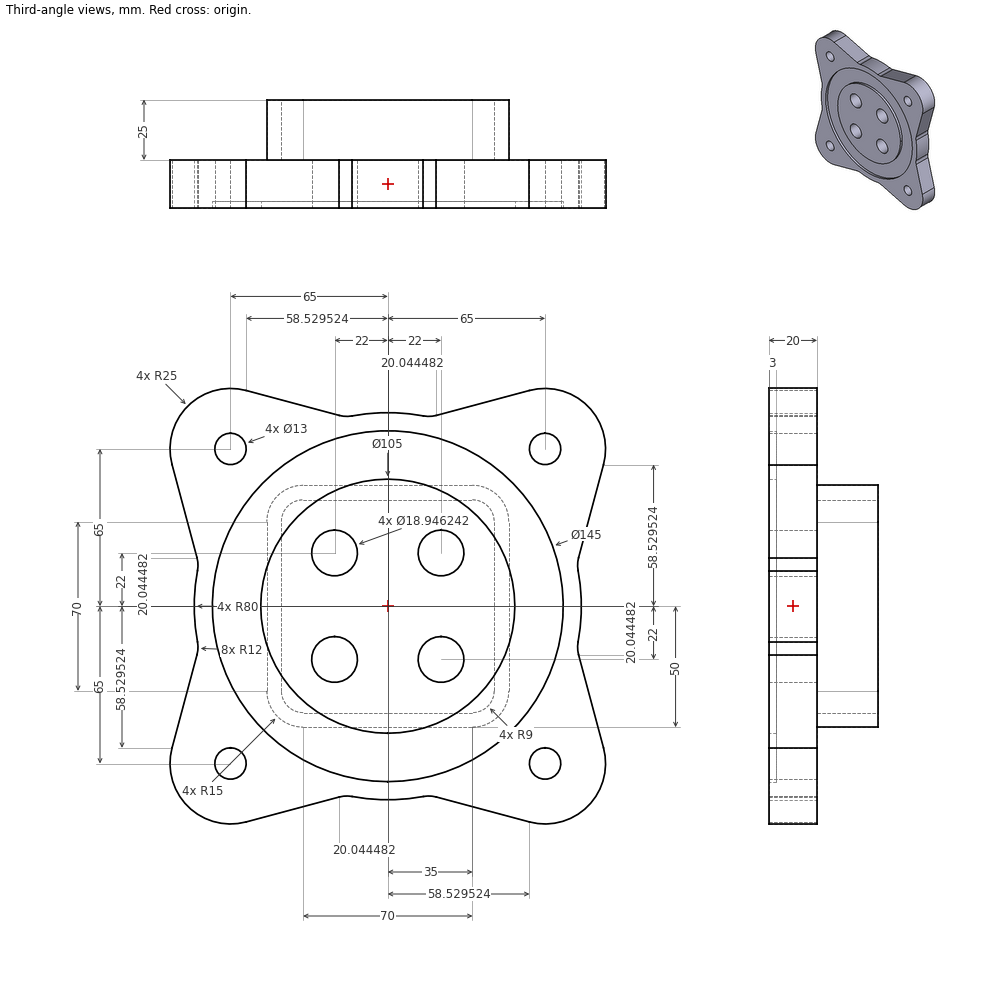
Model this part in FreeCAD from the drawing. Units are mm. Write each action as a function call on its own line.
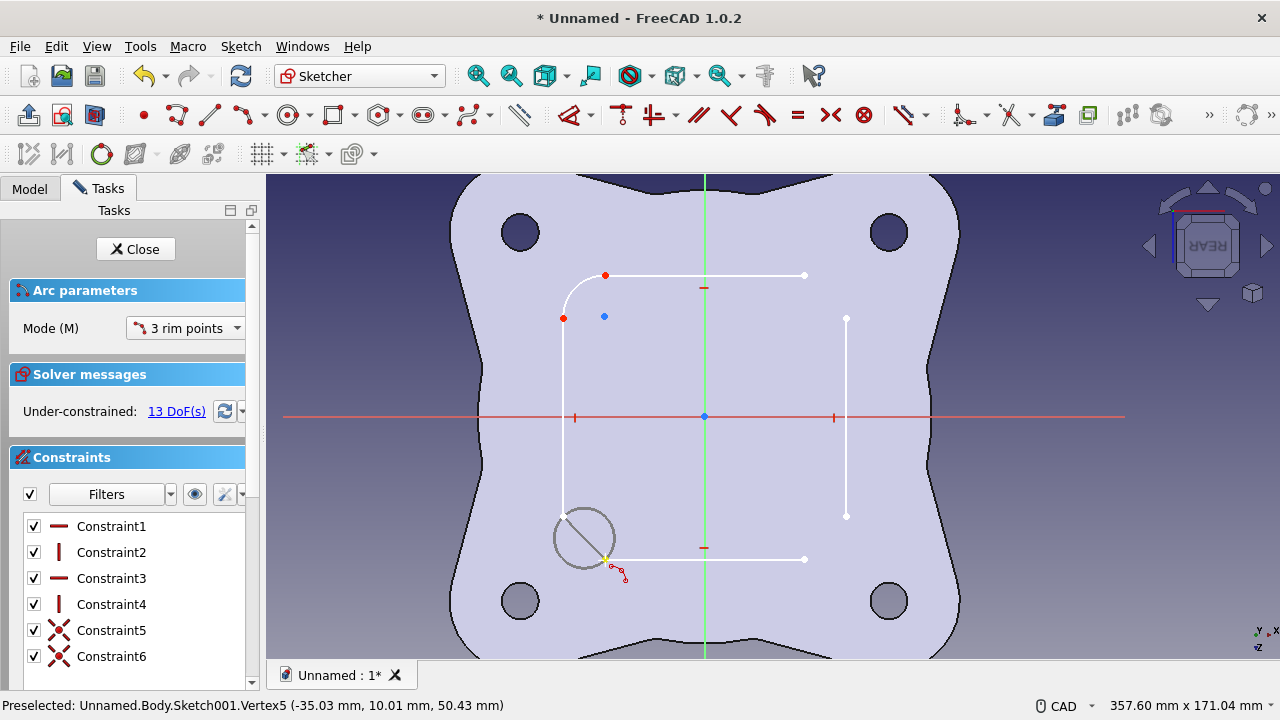
scroll(575, 546, up, 2)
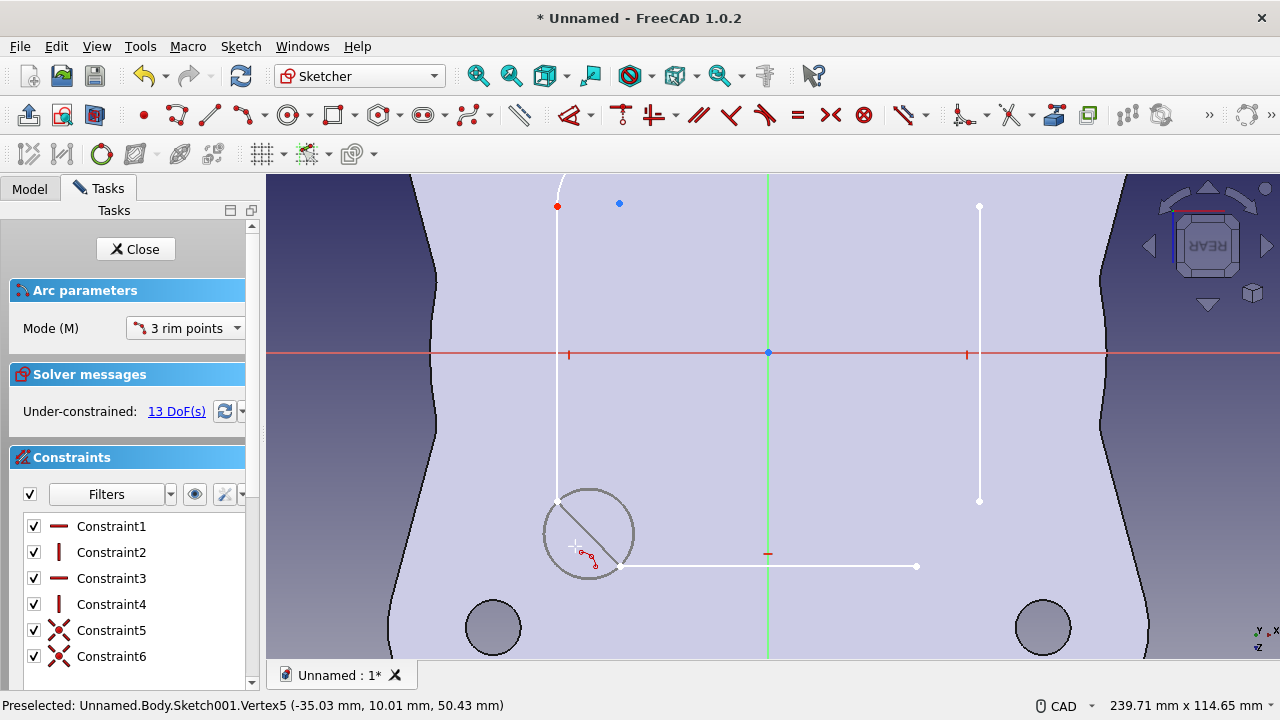
click(575, 546)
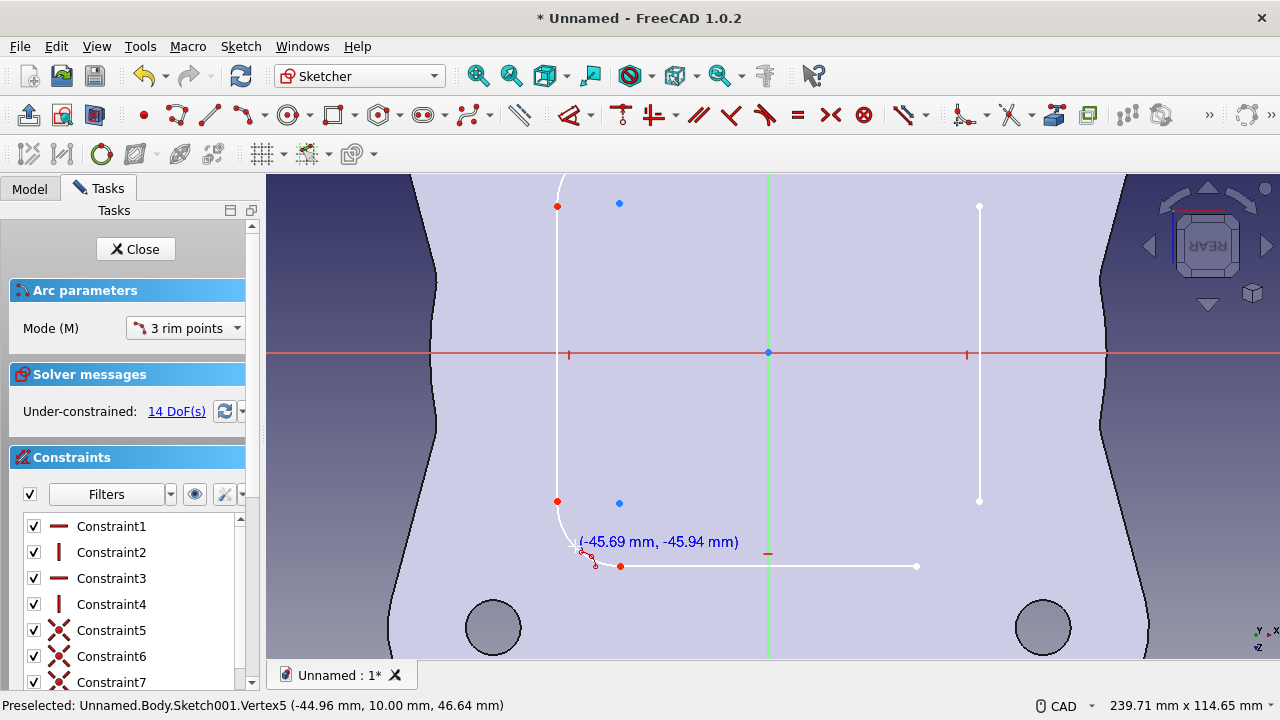
click(917, 566)
click(980, 502)
click(961, 546)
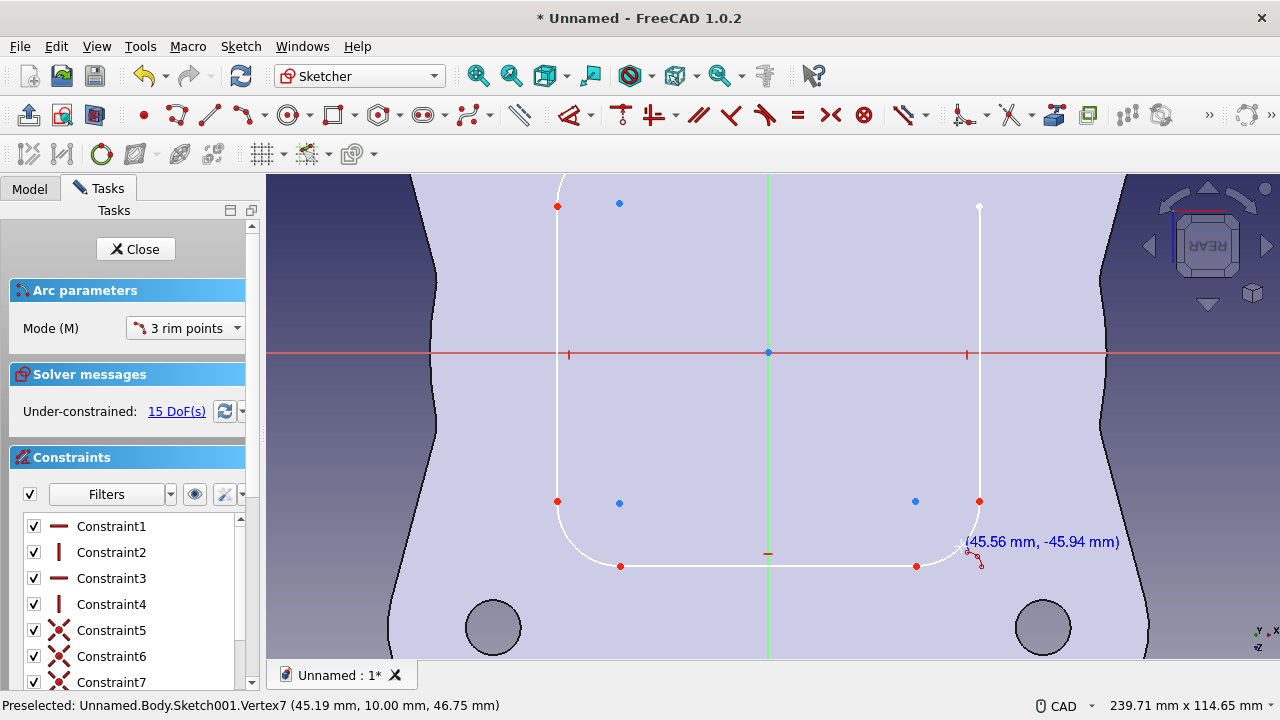
click(980, 206)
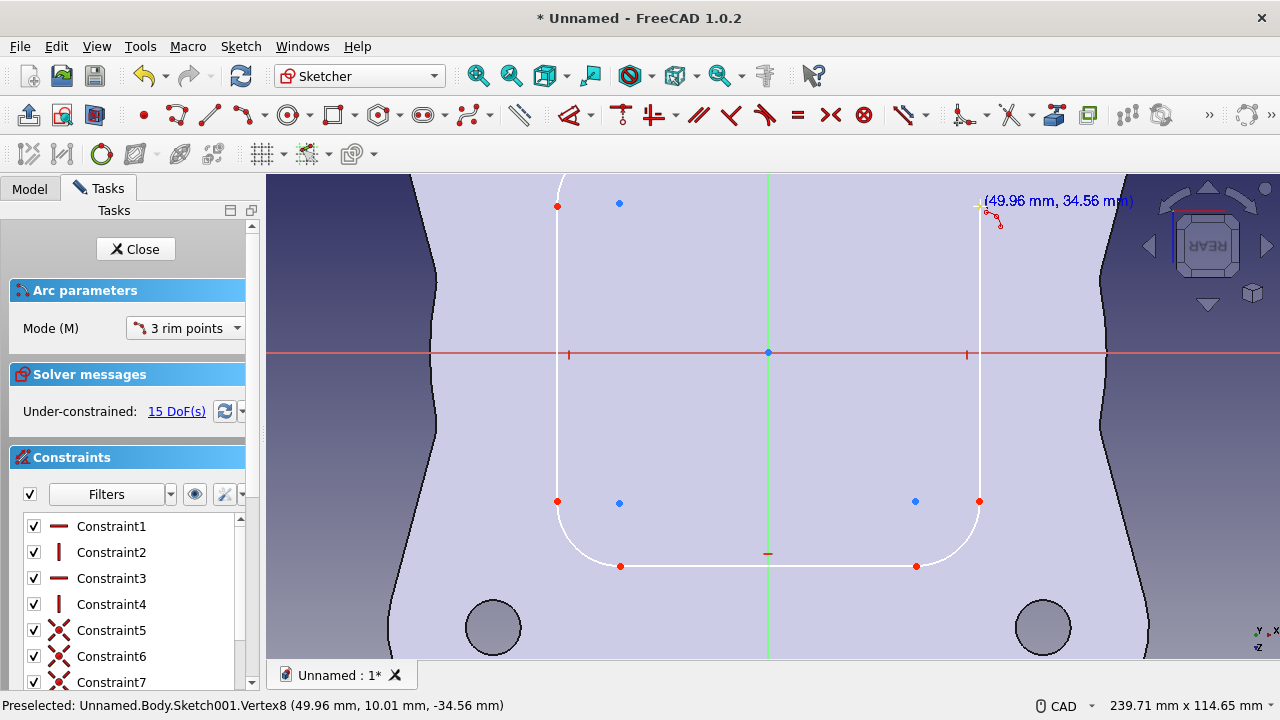
scroll(575, 546, down, 2)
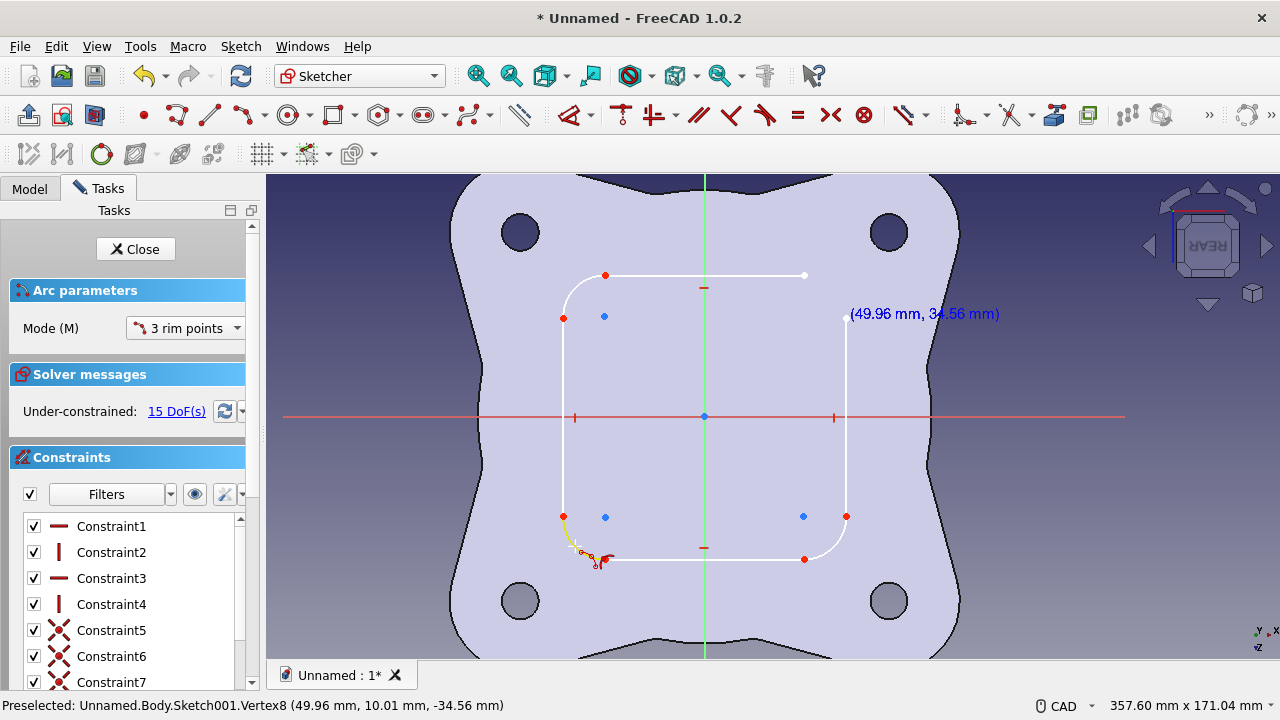
click(804, 276)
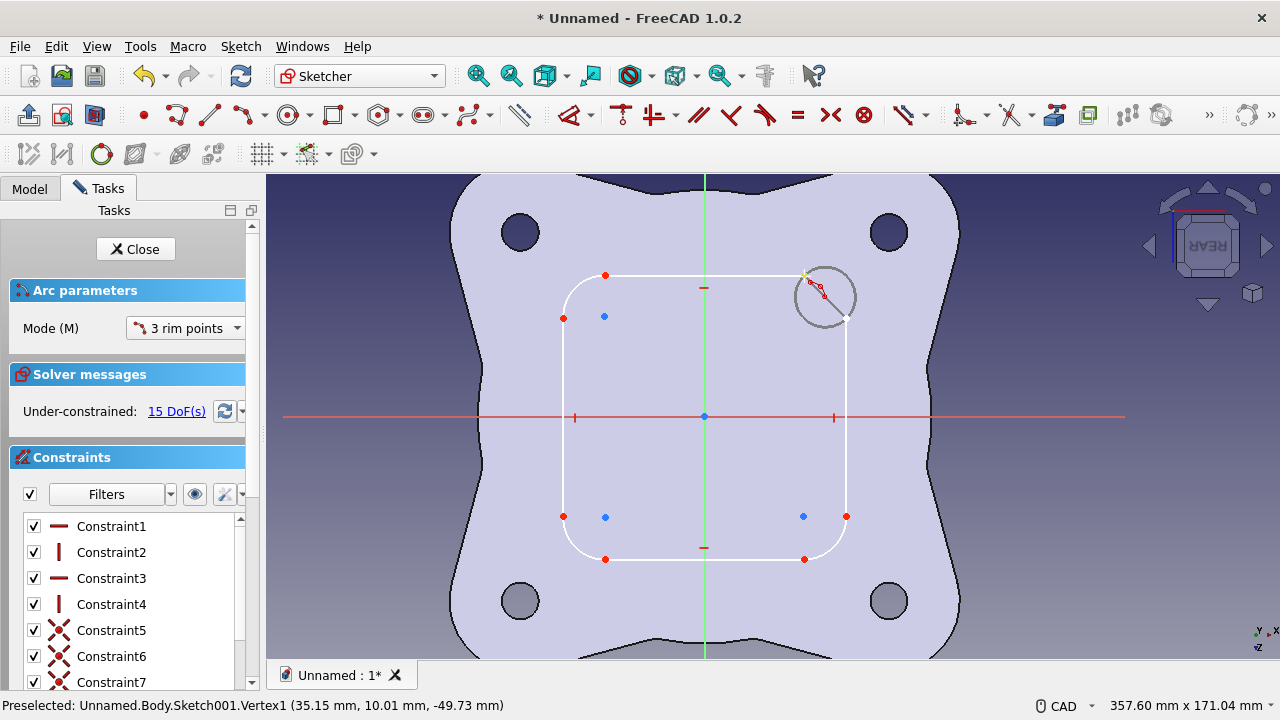
scroll(834, 287, up, 2)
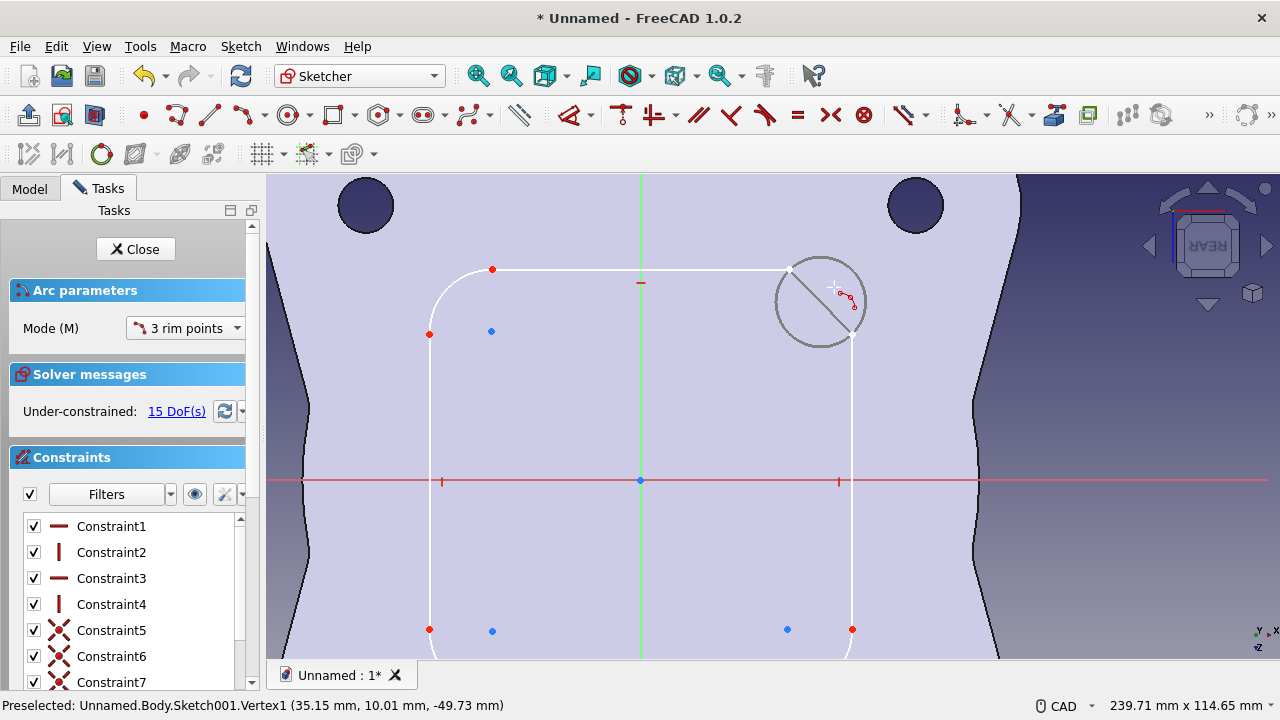
click(834, 287)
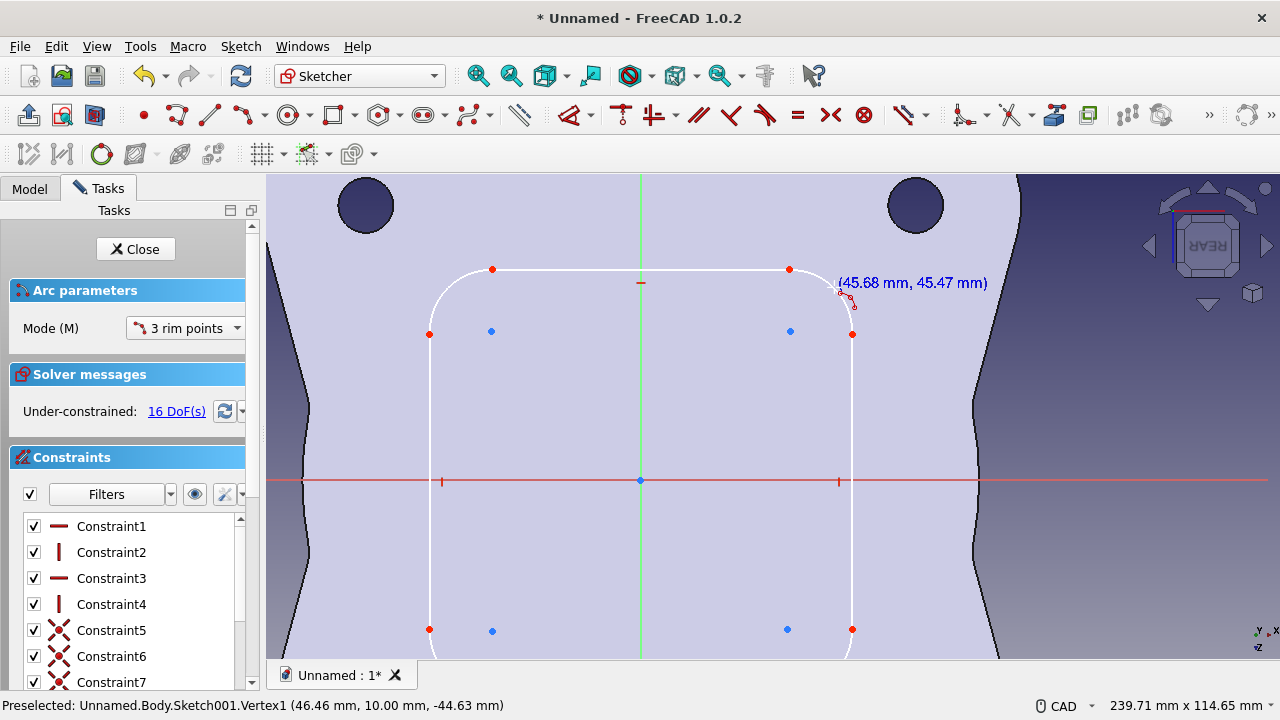
click(210, 116)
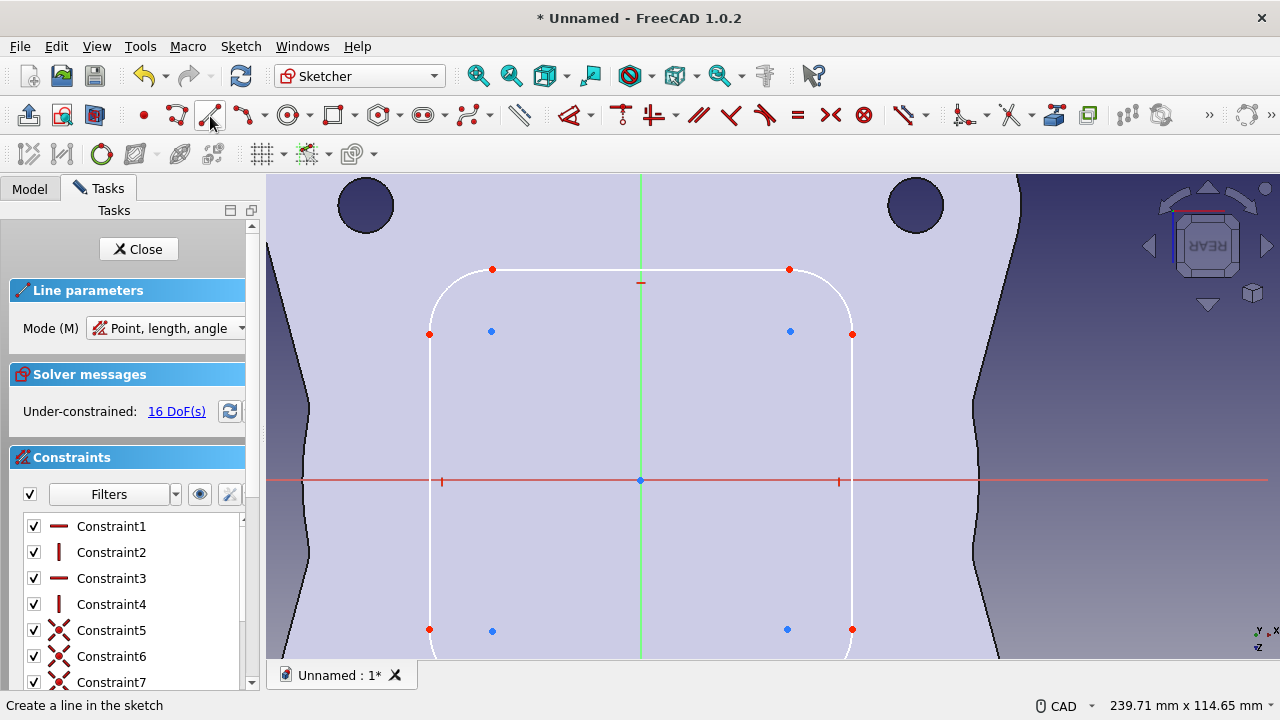
click(493, 294)
click(789, 294)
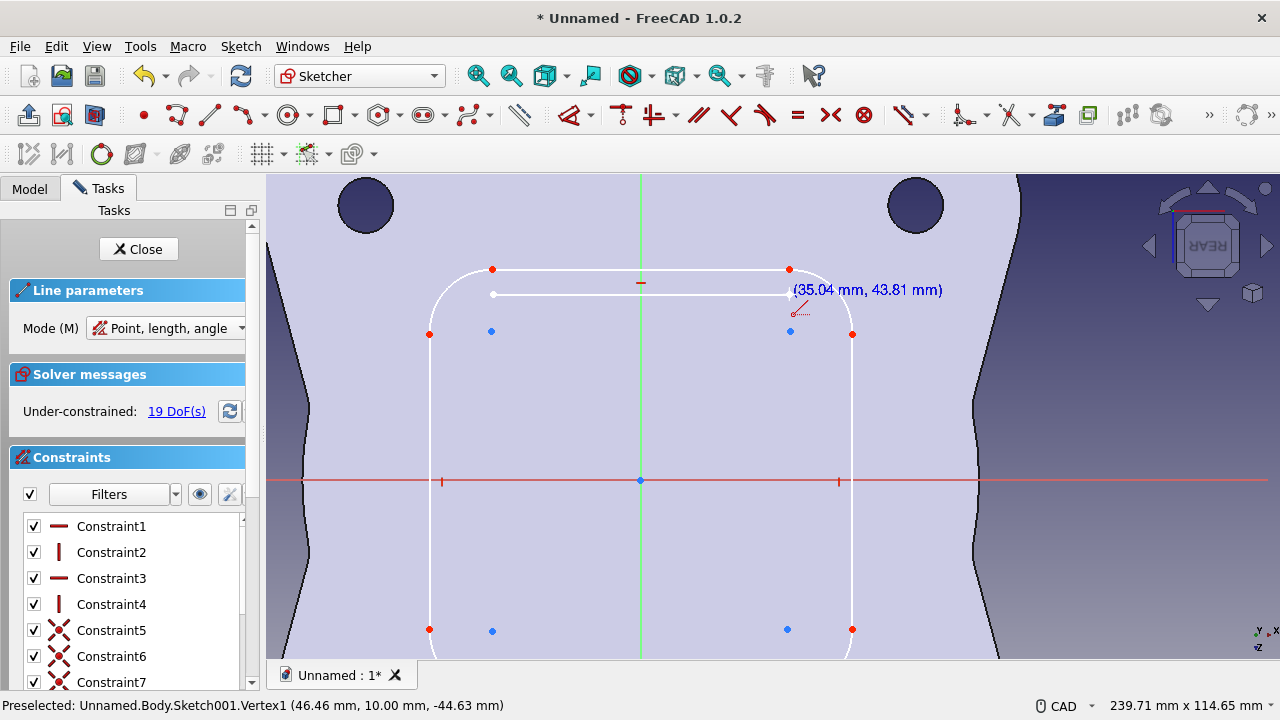
click(827, 332)
click(827, 628)